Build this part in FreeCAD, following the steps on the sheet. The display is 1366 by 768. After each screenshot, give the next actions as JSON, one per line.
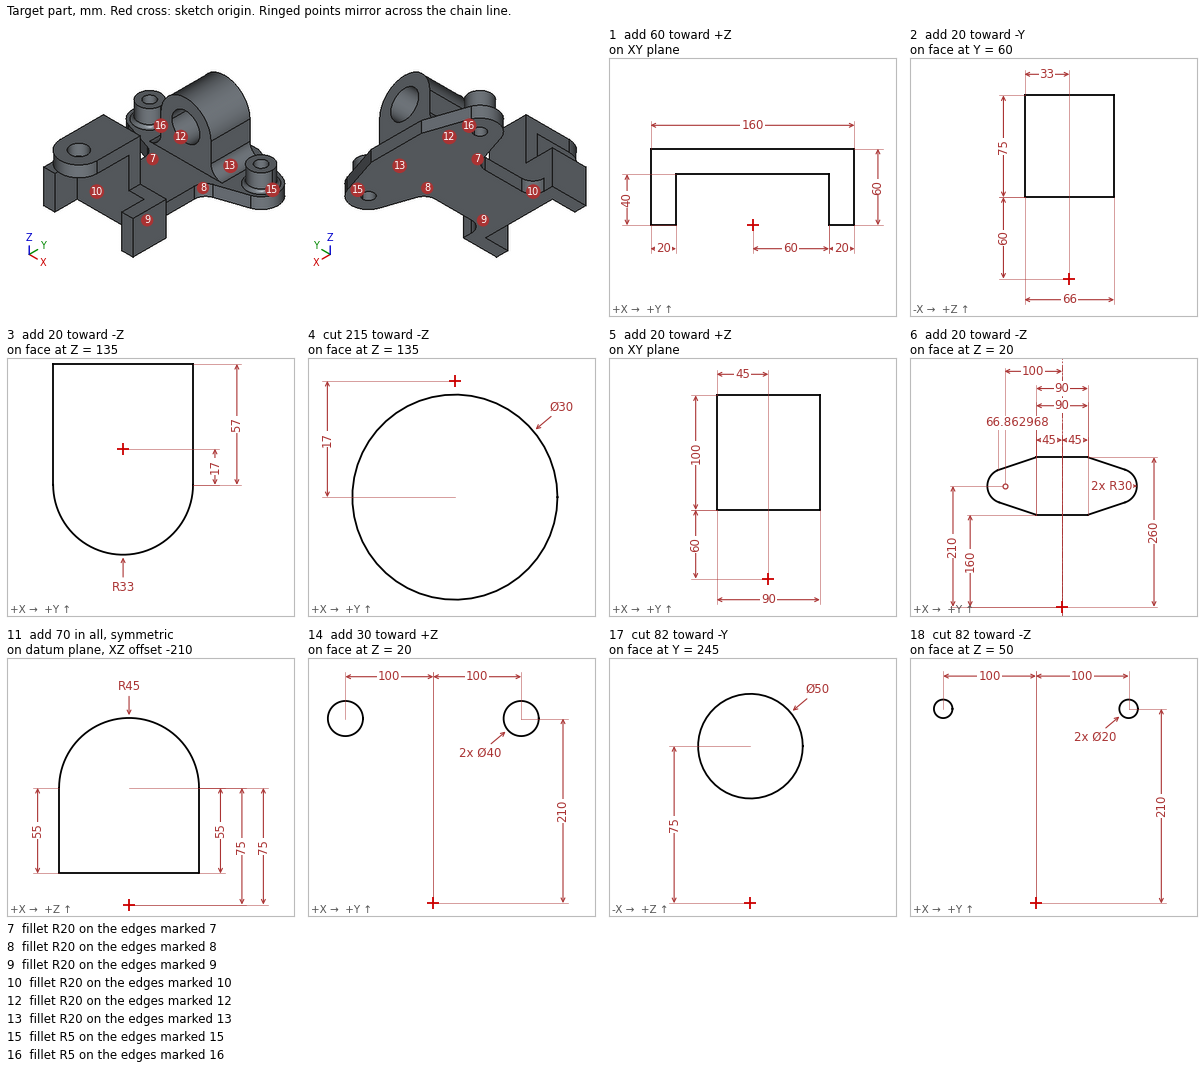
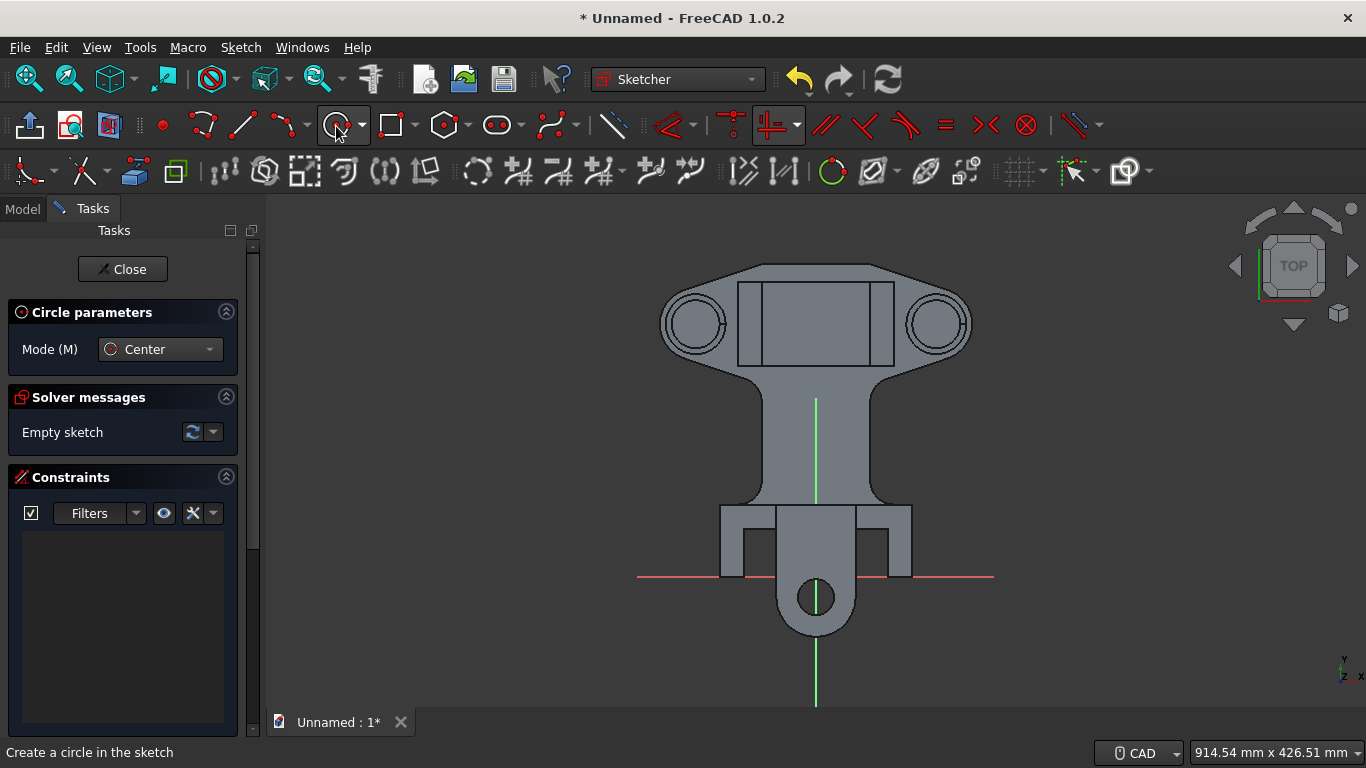
{"action": "scroll", "coordinate": [936, 324], "scroll_direction": "up", "scroll_amount": 4}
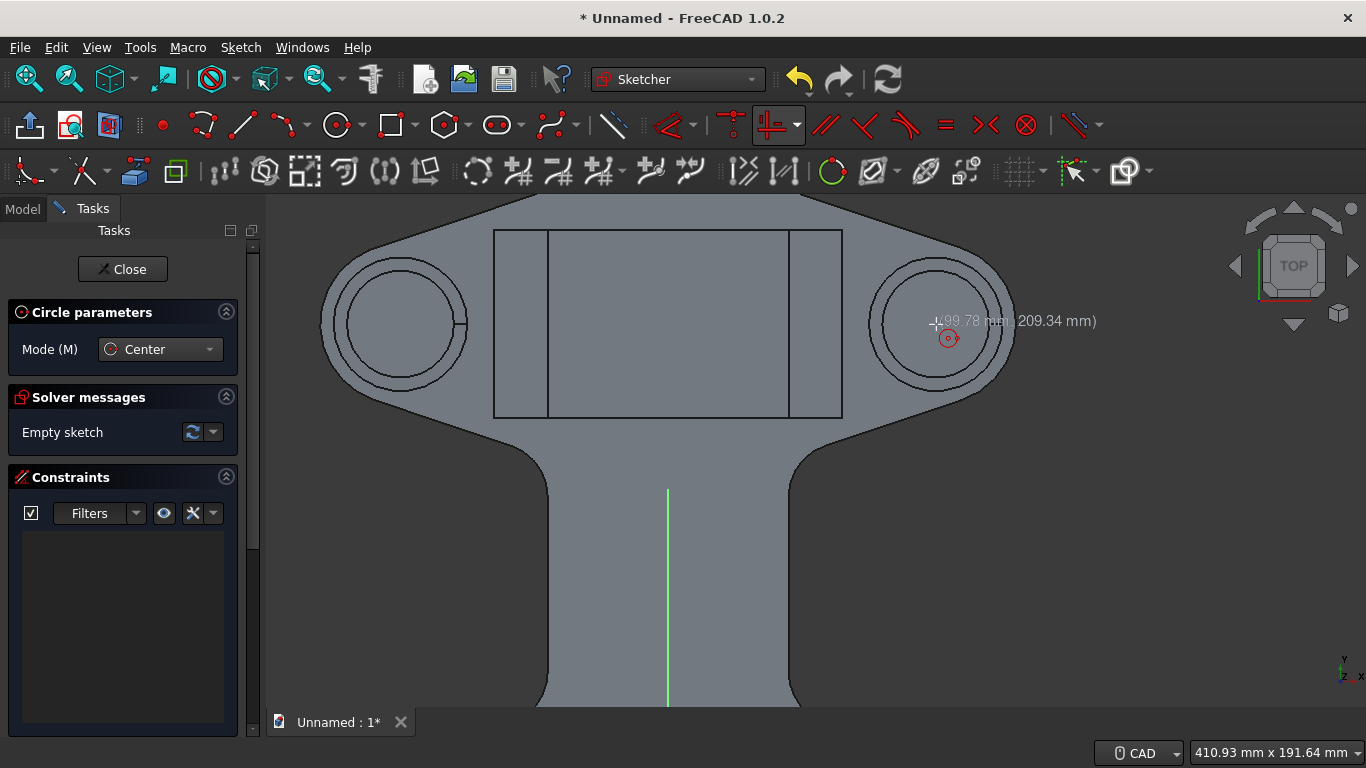
{"action": "left_click", "coordinate": [936, 324]}
{"action": "left_click", "coordinate": [955, 305]}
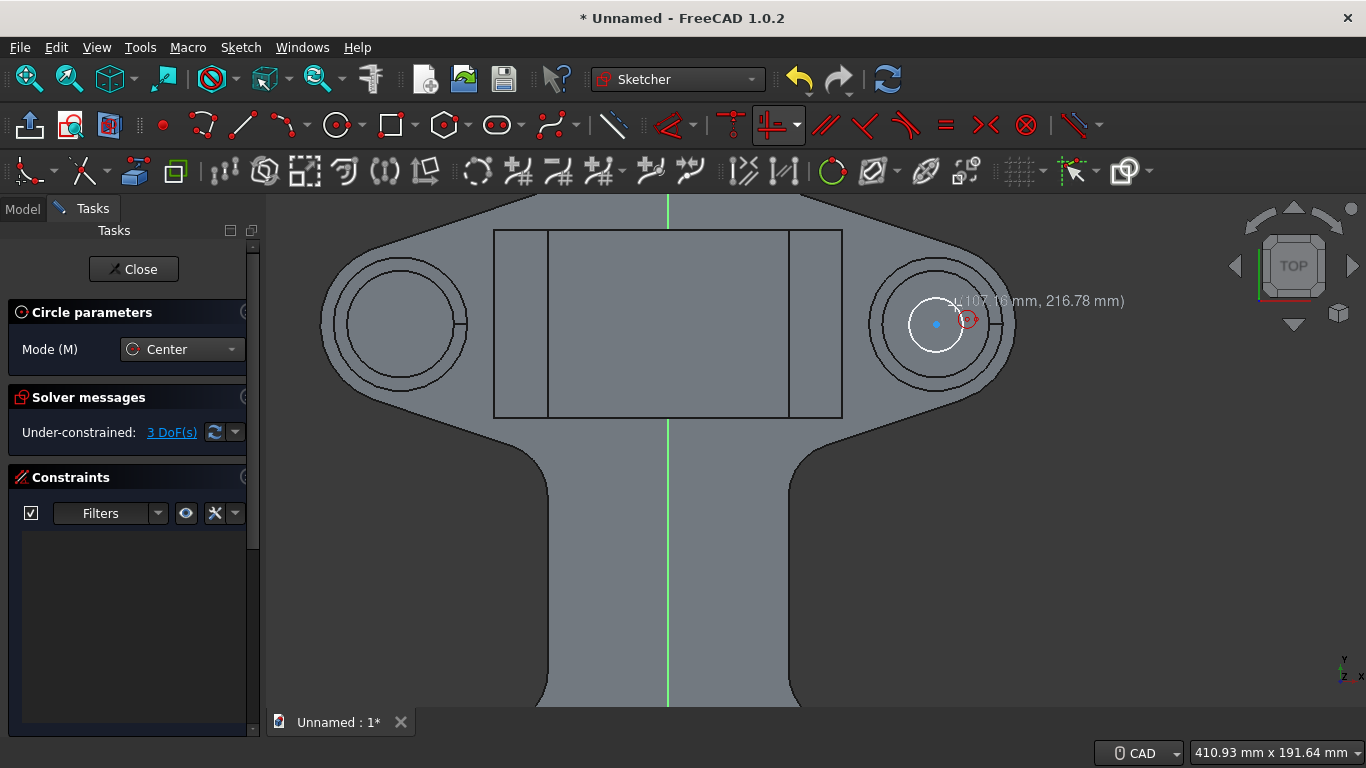
{"action": "left_click", "coordinate": [400, 324]}
{"action": "left_click", "coordinate": [419, 305]}
{"action": "key", "text": "Escape"}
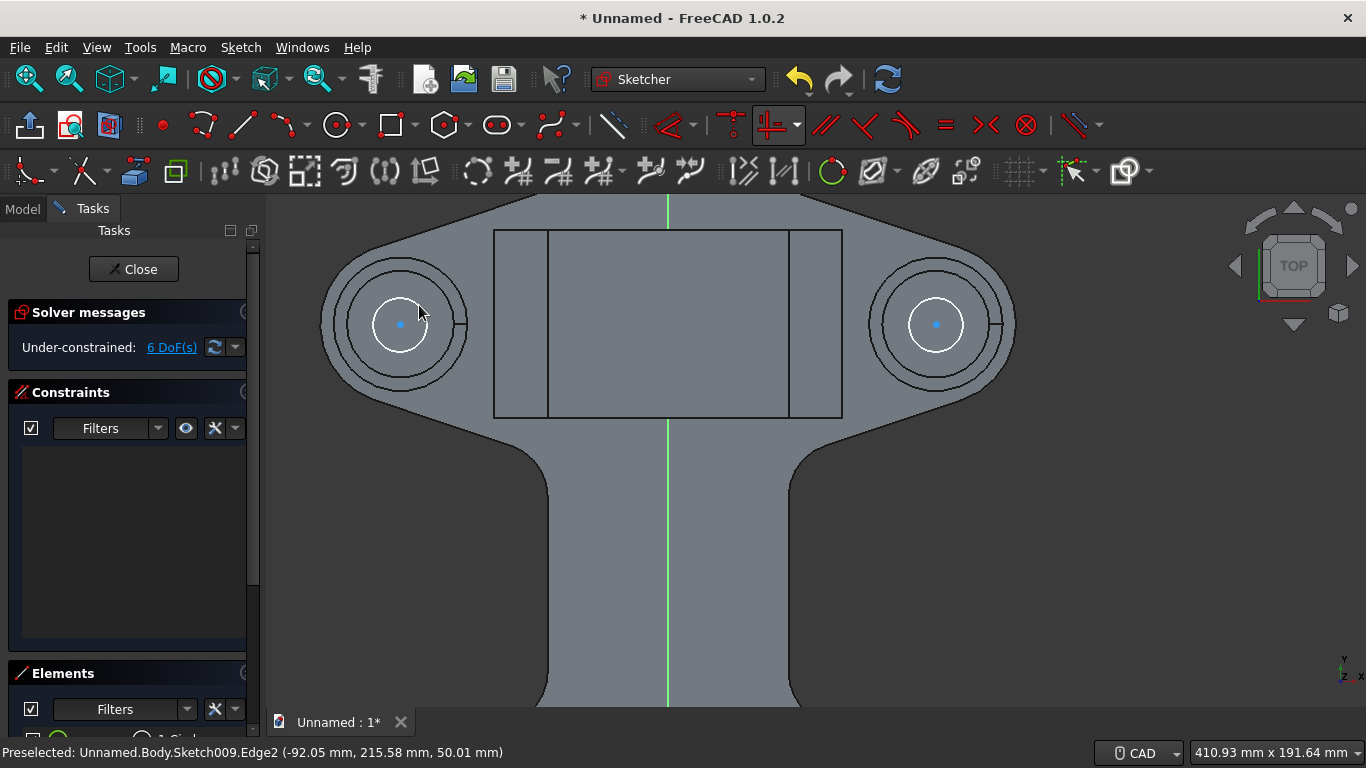
{"action": "left_click", "coordinate": [955, 306]}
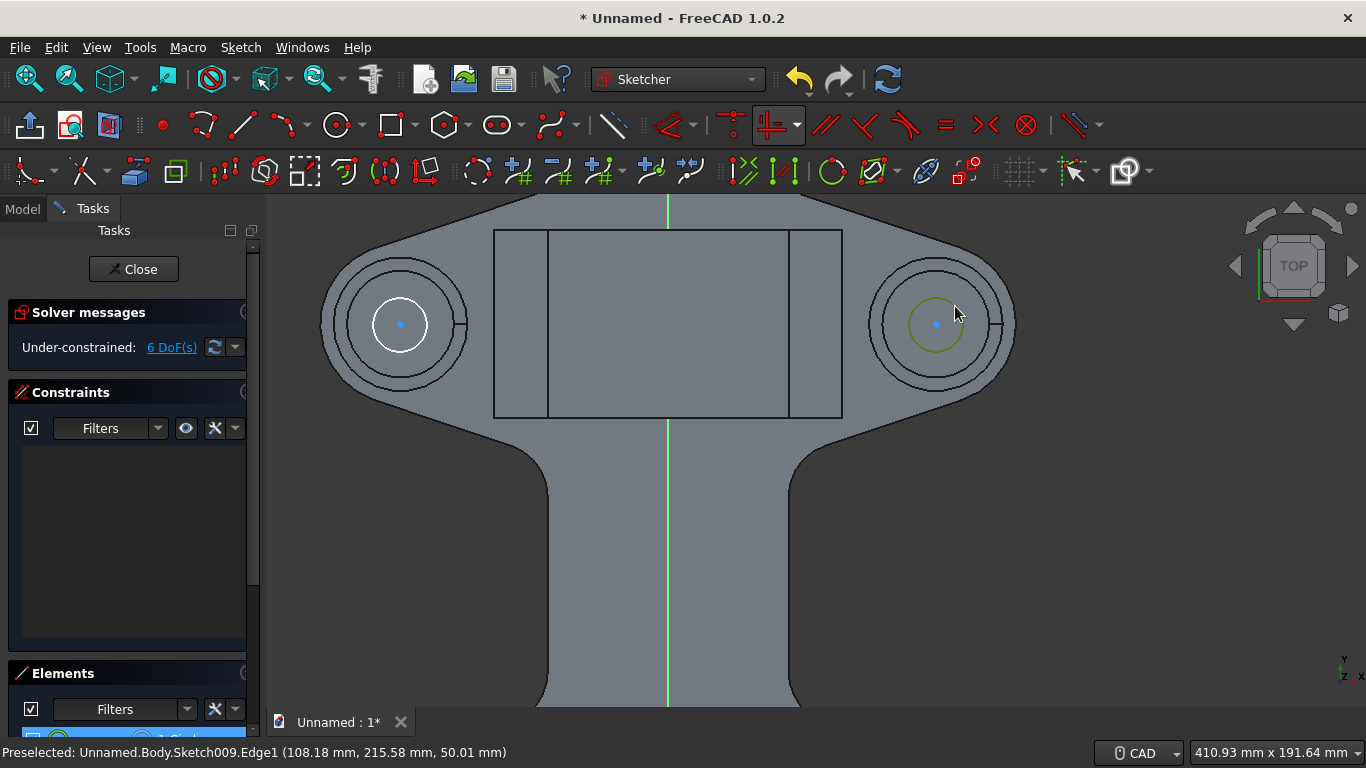
{"action": "left_click", "coordinate": [419, 306]}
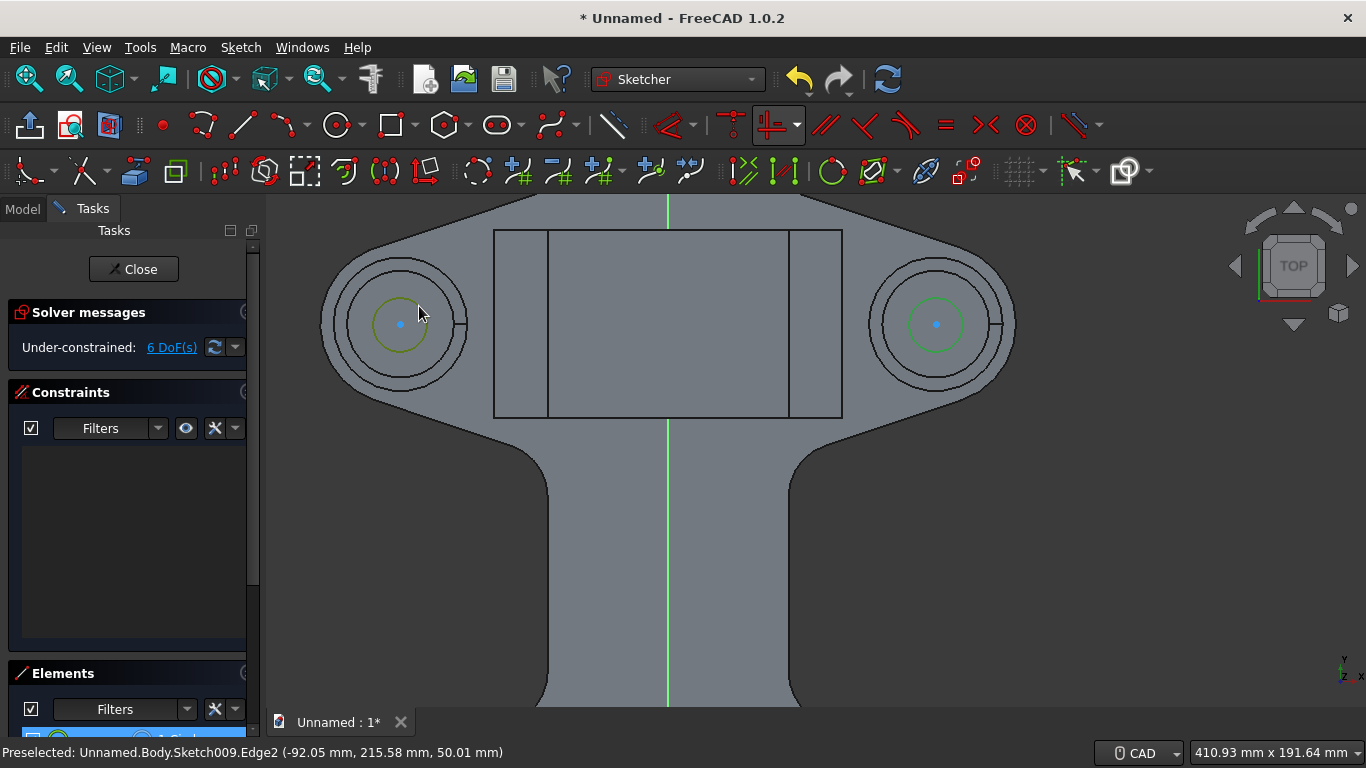
{"action": "key", "text": "e"}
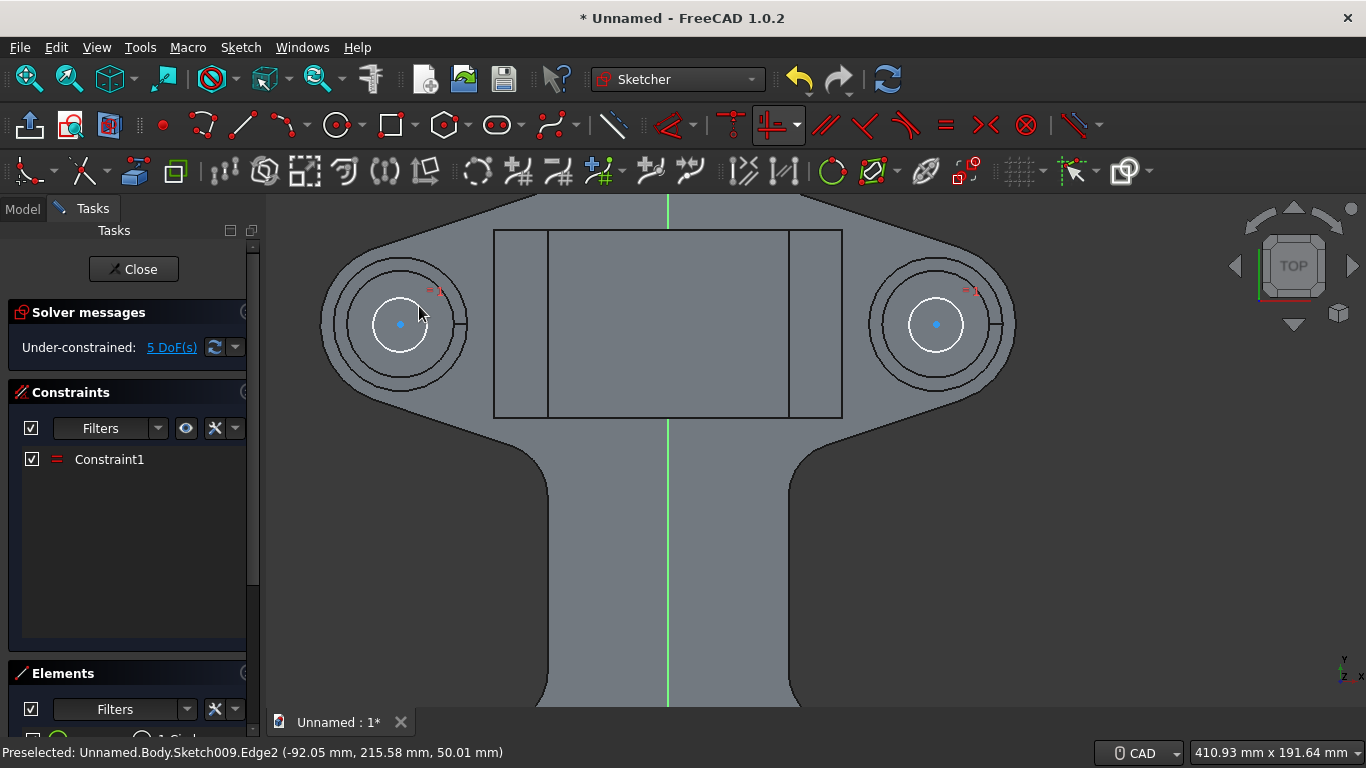
{"action": "left_click", "coordinate": [936, 325]}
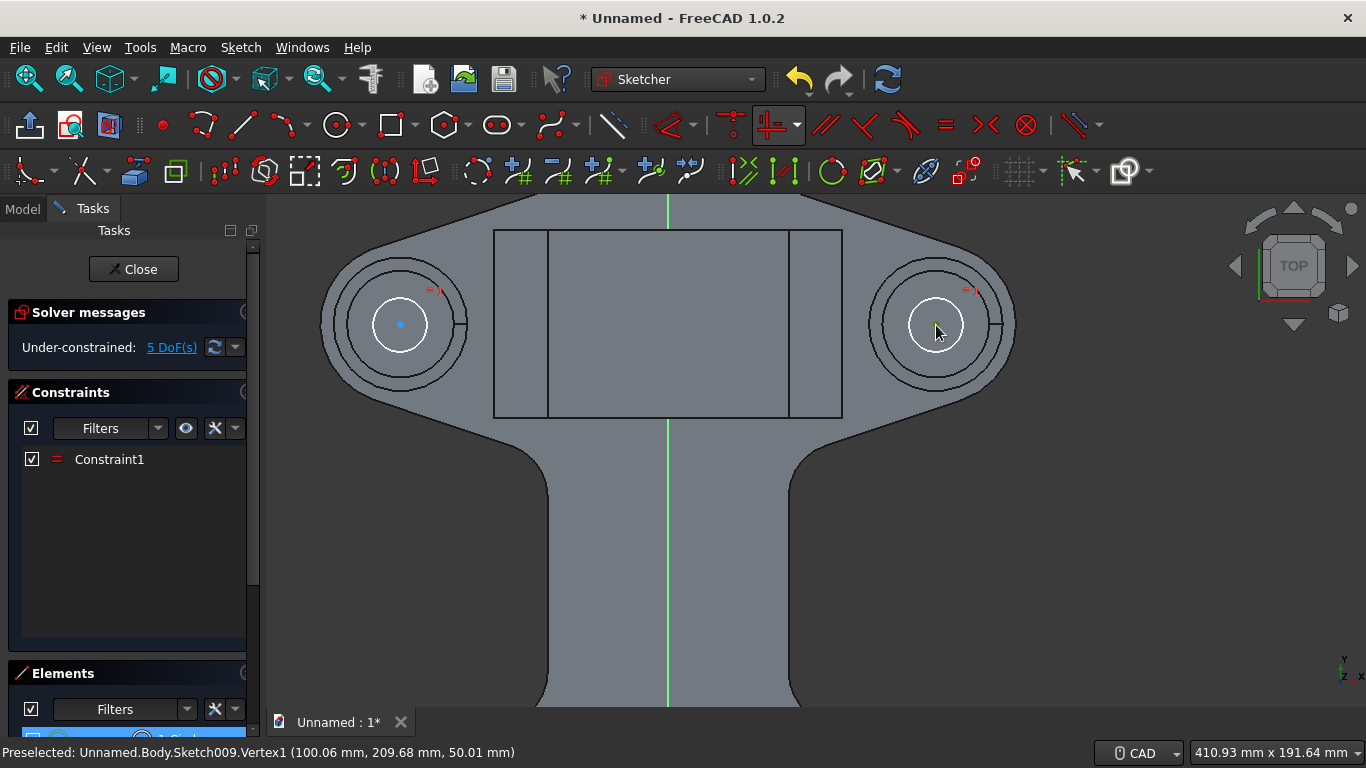
{"action": "left_click", "coordinate": [400, 325]}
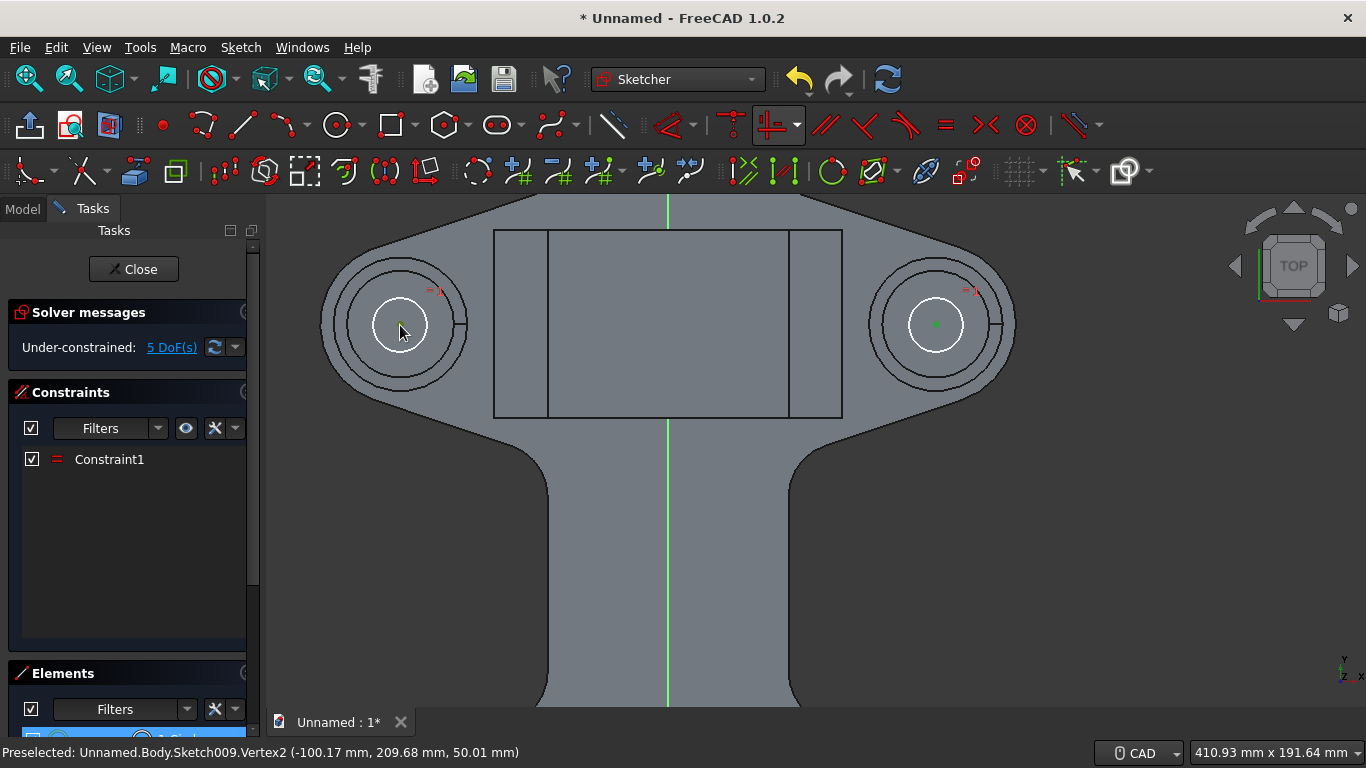
{"action": "key", "text": "h"}